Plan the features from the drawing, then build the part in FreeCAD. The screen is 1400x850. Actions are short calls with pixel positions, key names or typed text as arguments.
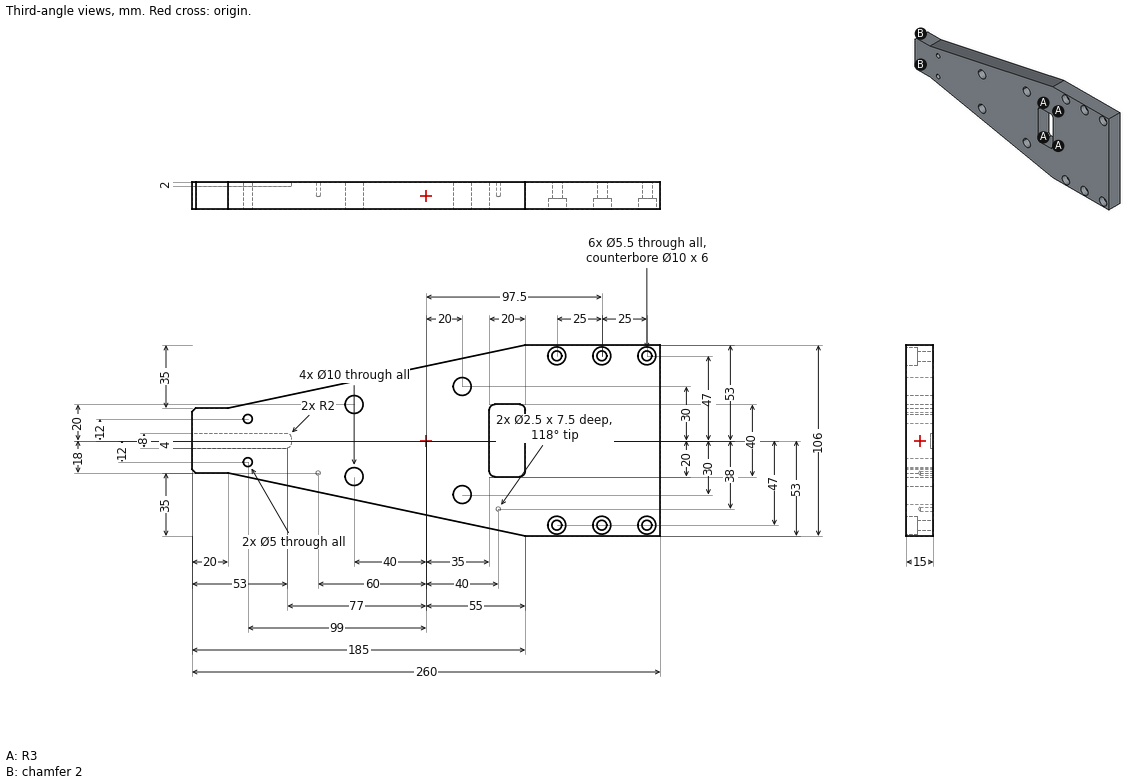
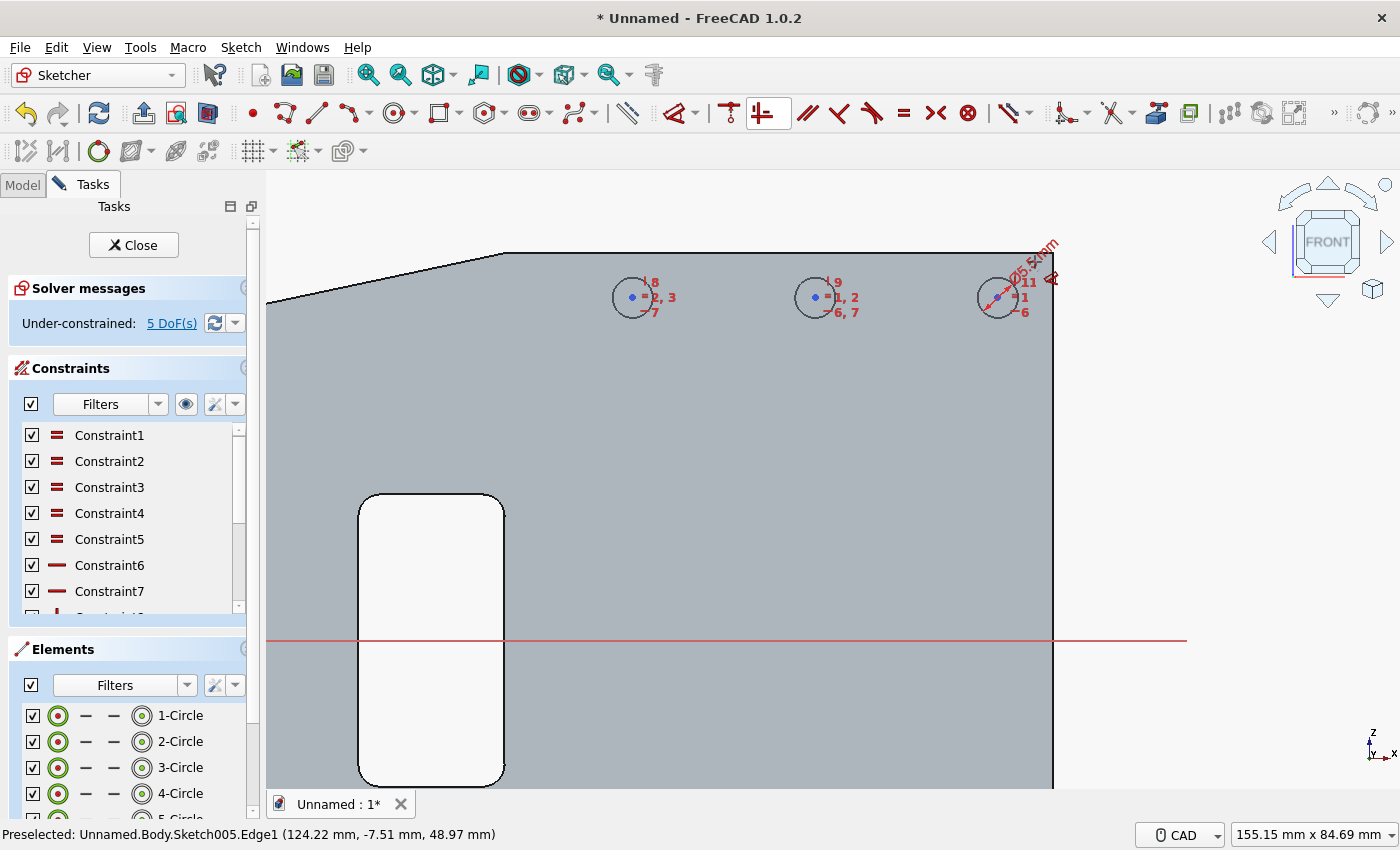
click(998, 298)
click(1032, 469)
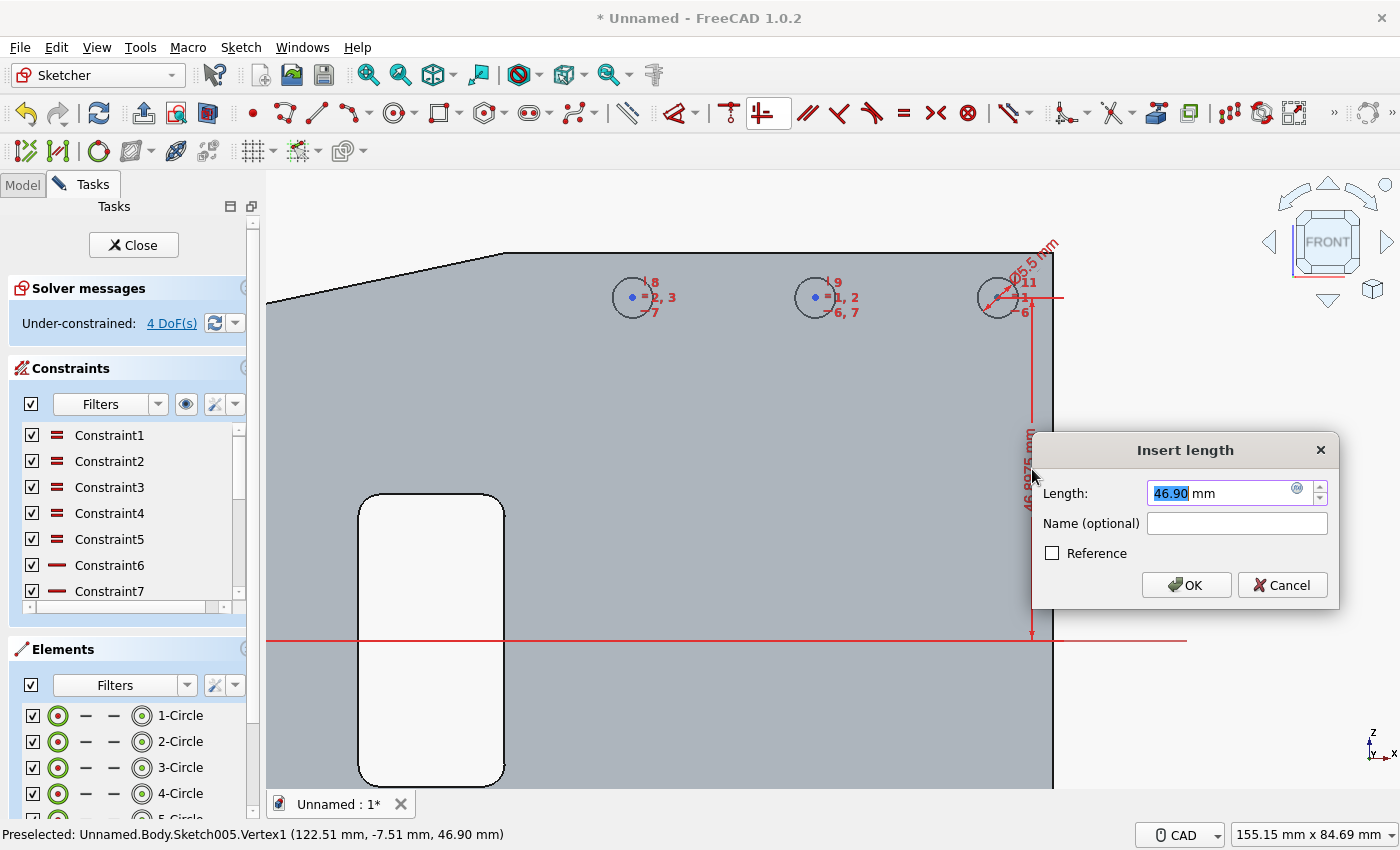
text(47)
key(Return)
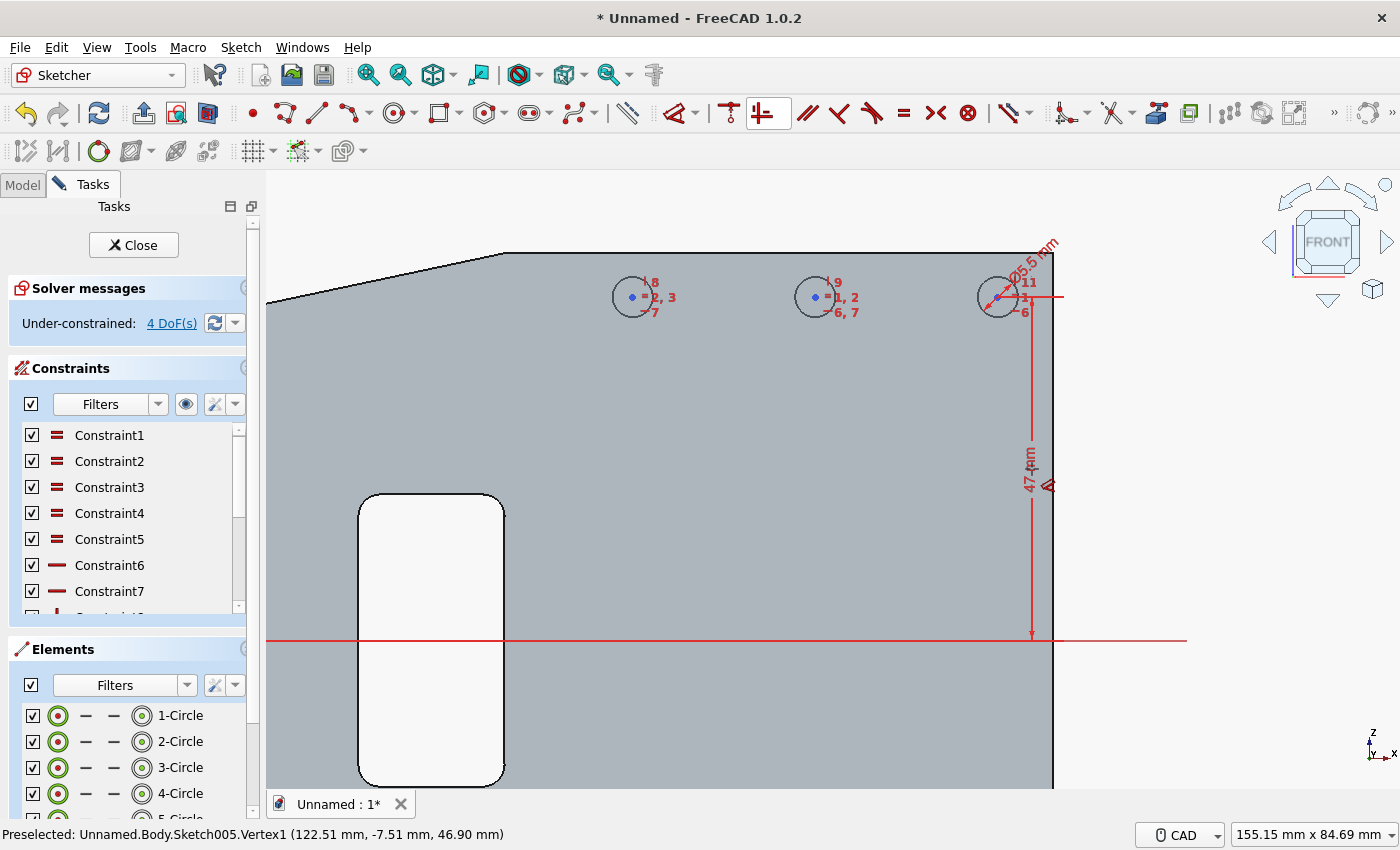
scroll(1013, 284, down, 3)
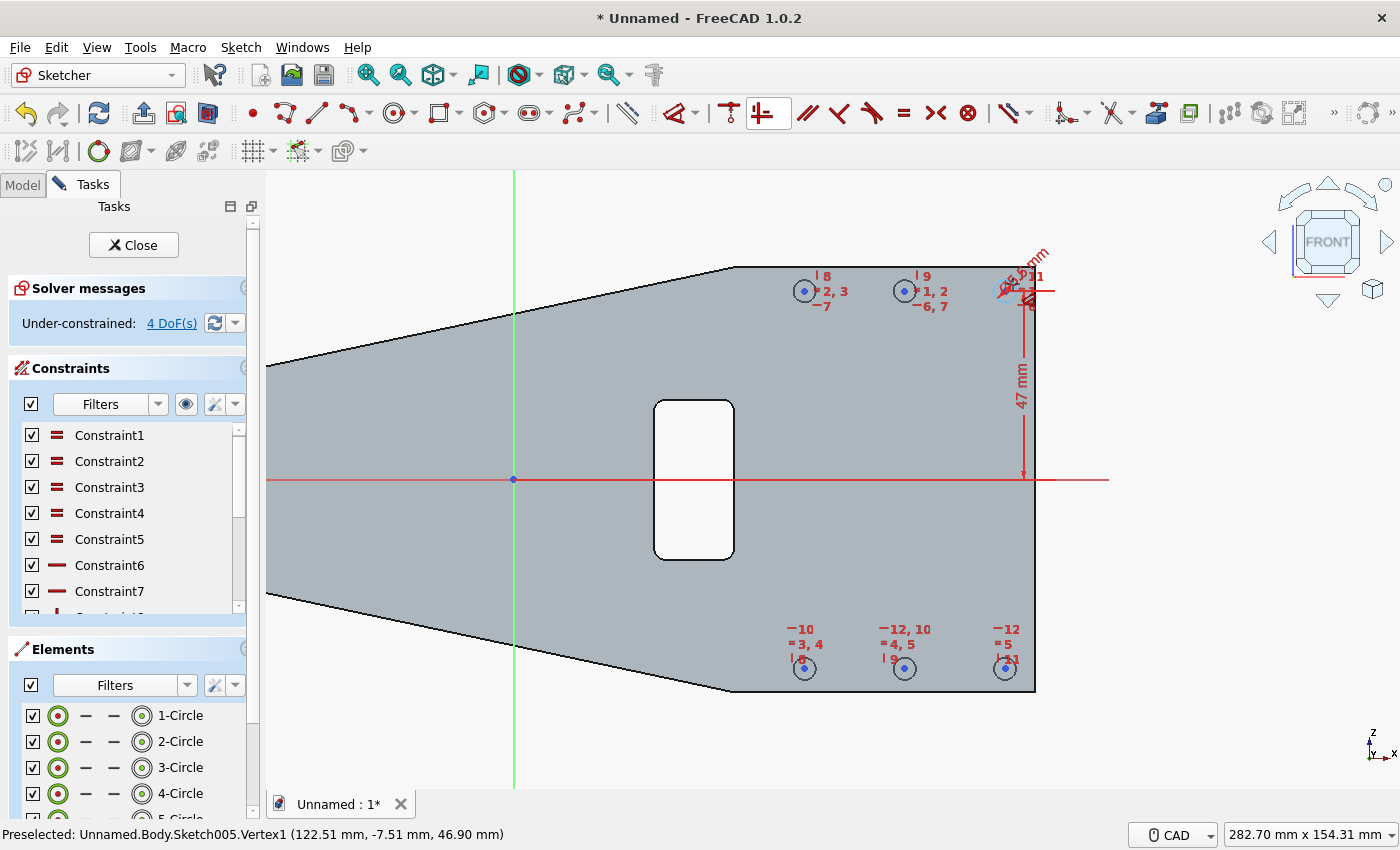
click(805, 669)
click(480, 574)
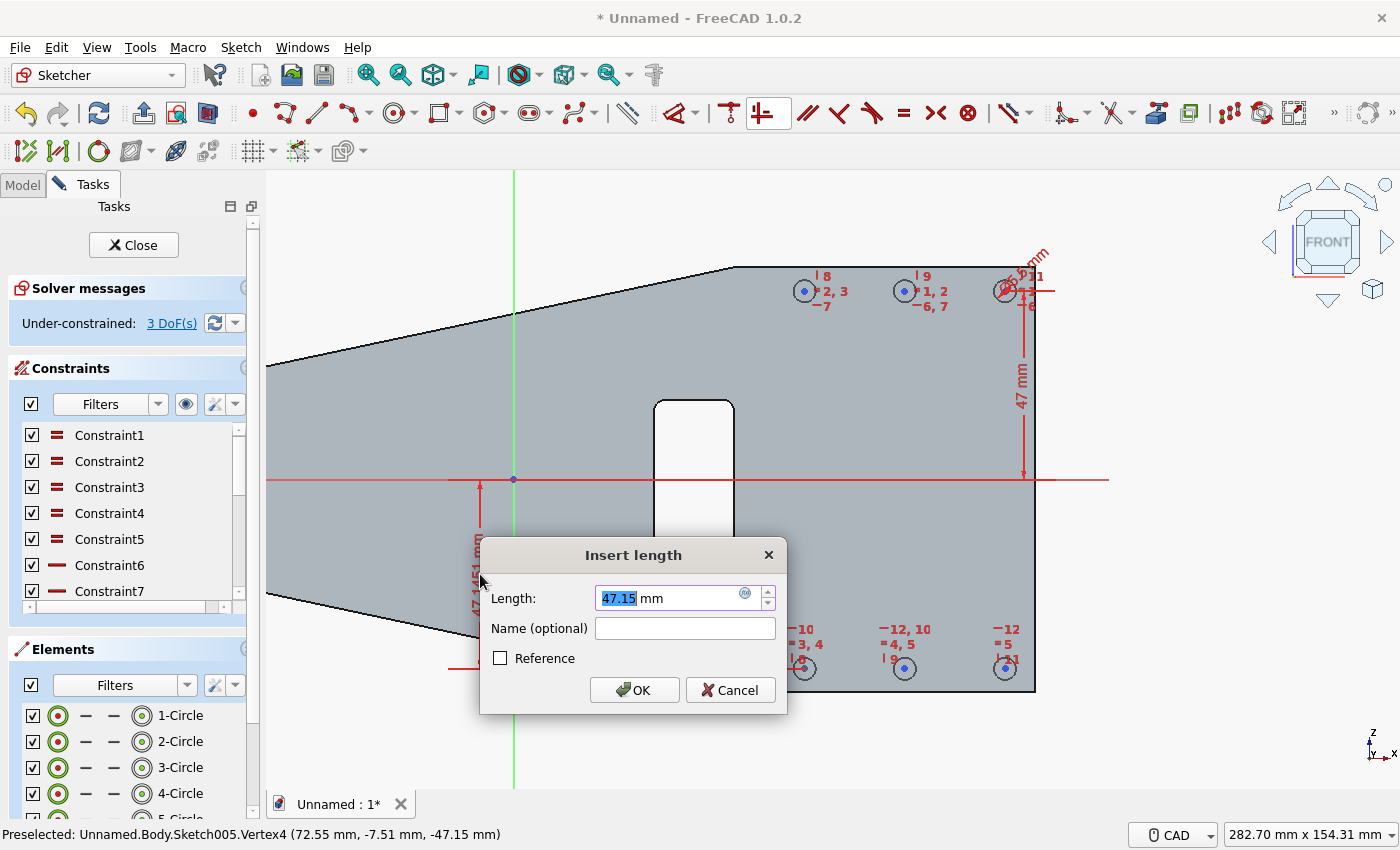
text(47)
key(Return)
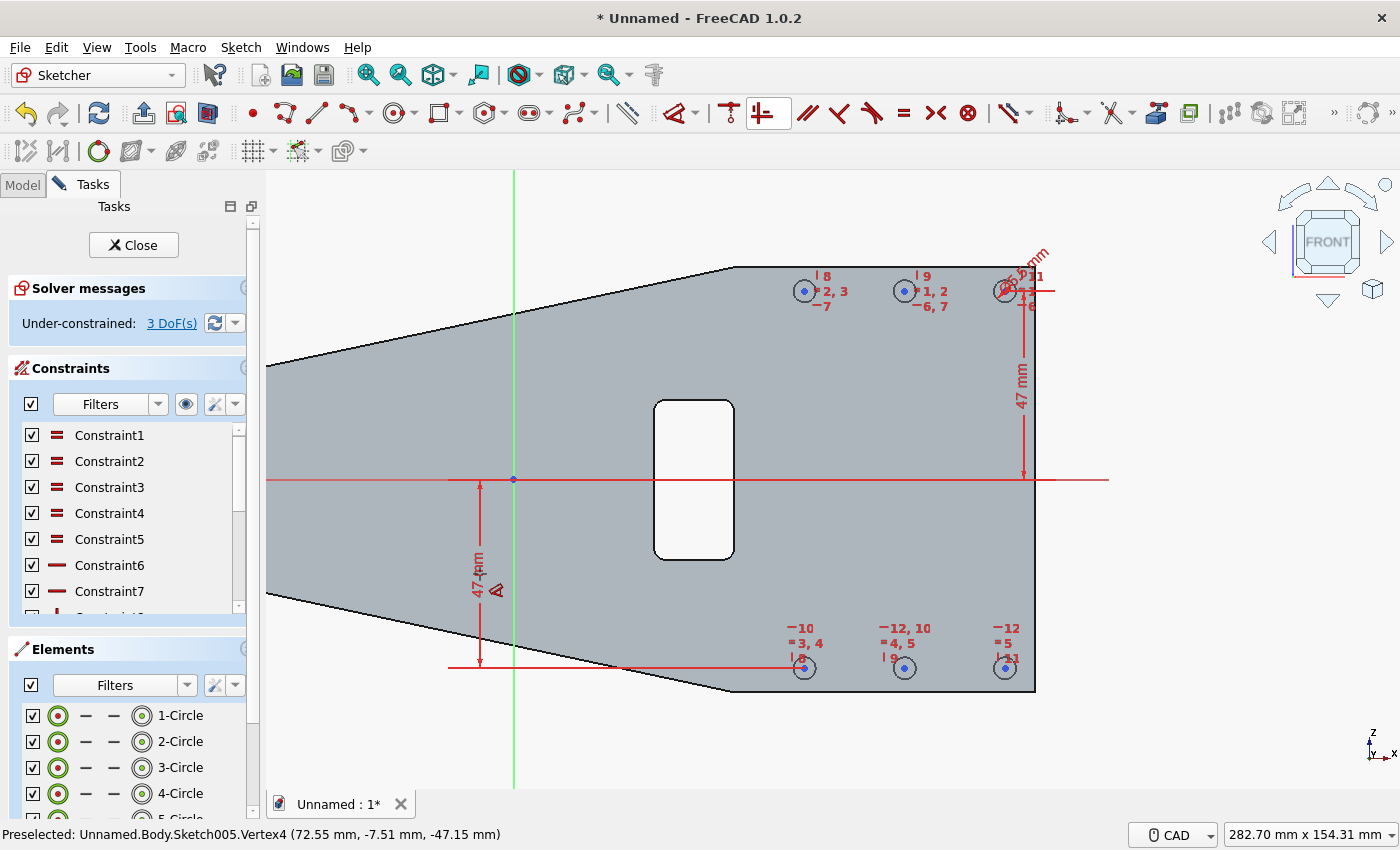
click(1005, 291)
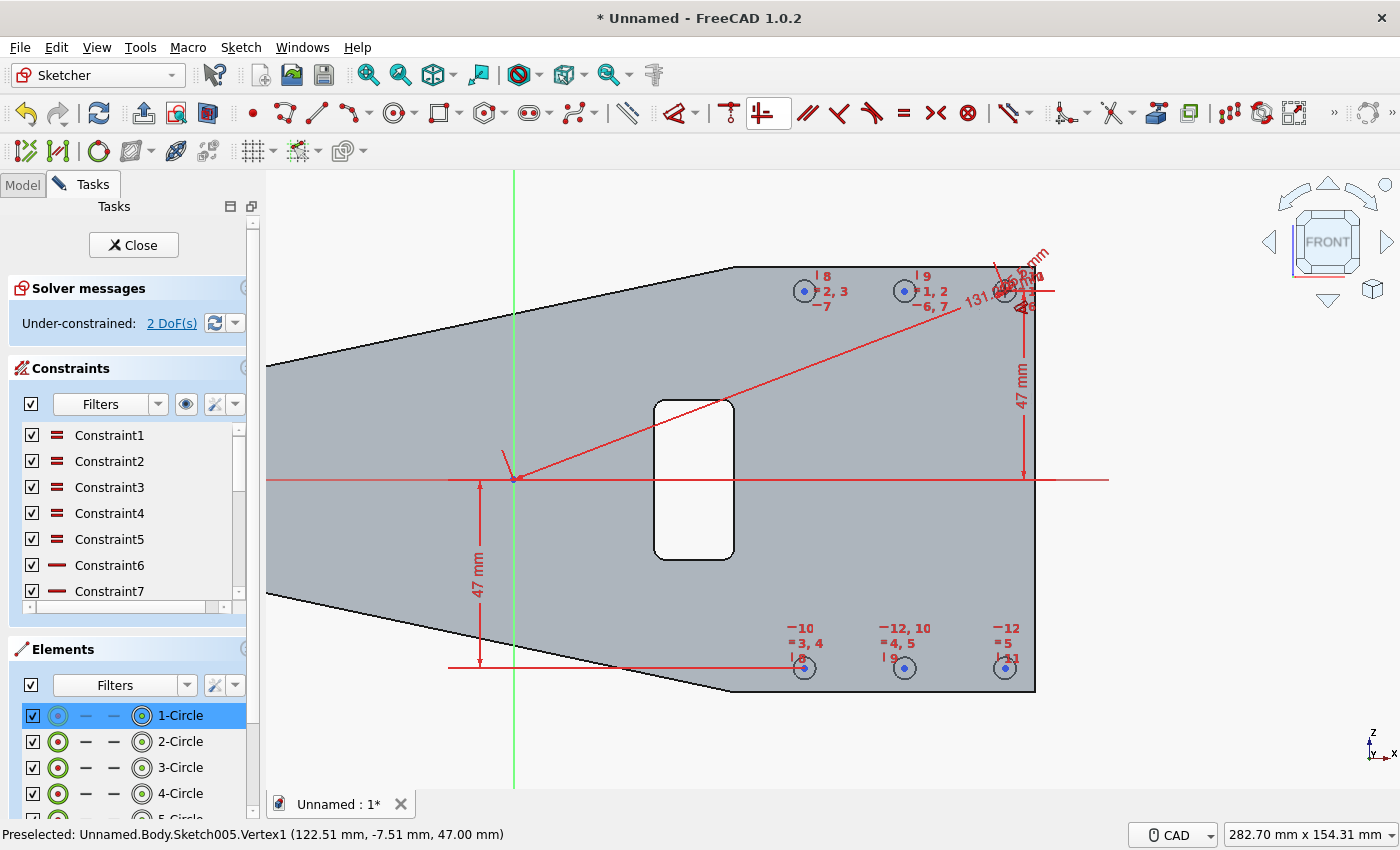
click(905, 291)
click(955, 257)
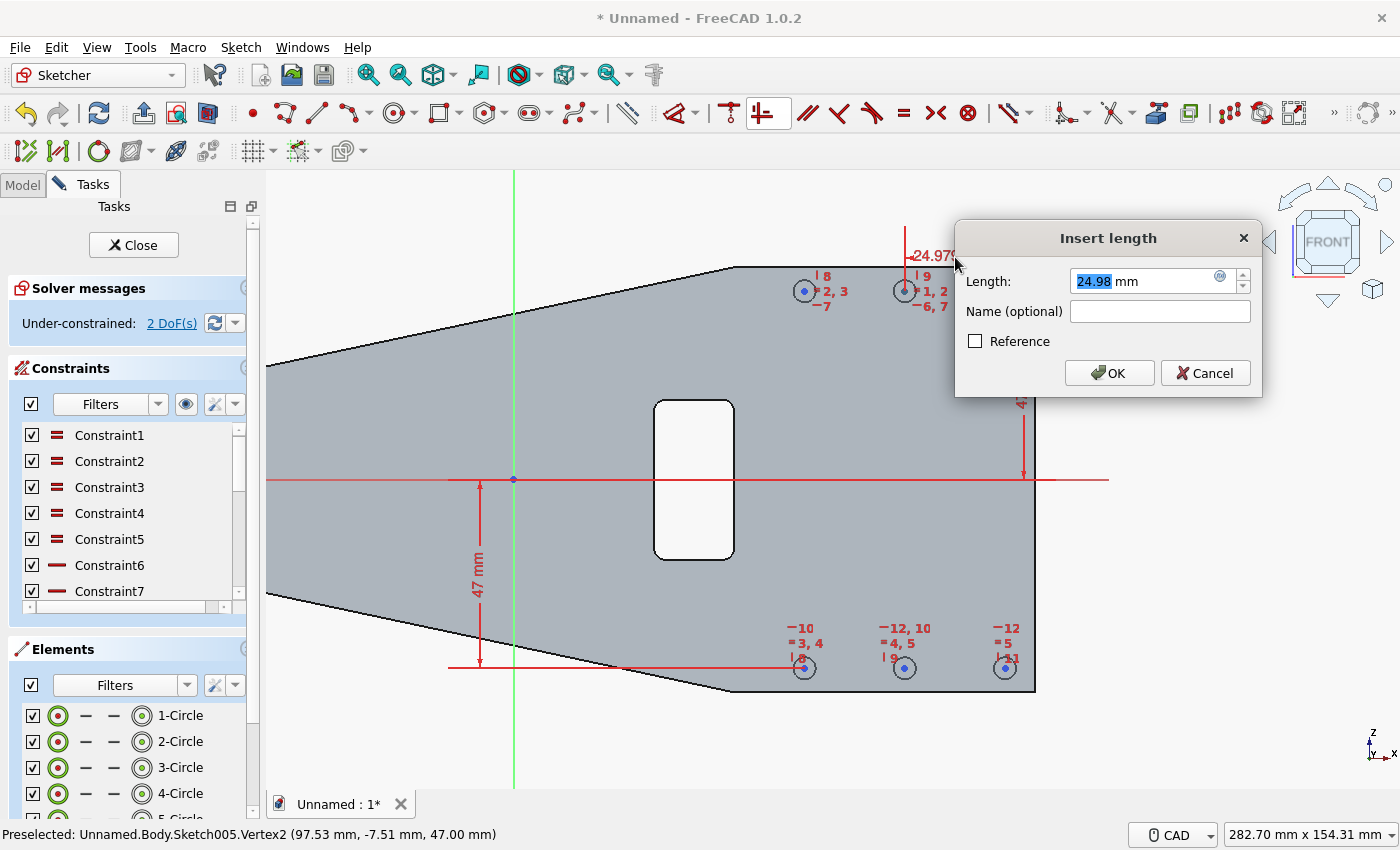
text(25)
key(Return)